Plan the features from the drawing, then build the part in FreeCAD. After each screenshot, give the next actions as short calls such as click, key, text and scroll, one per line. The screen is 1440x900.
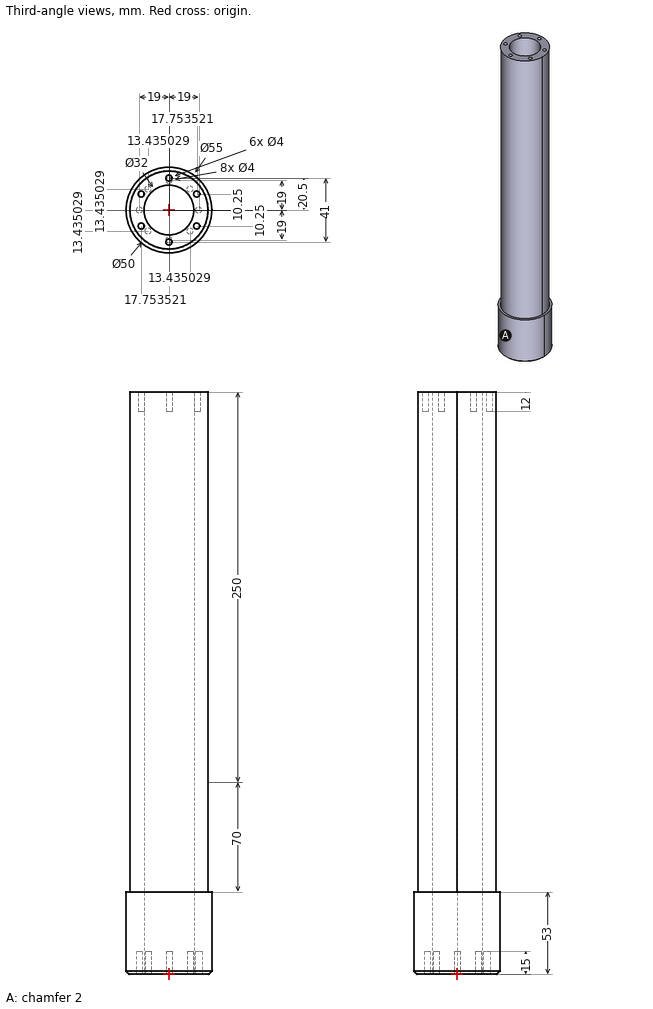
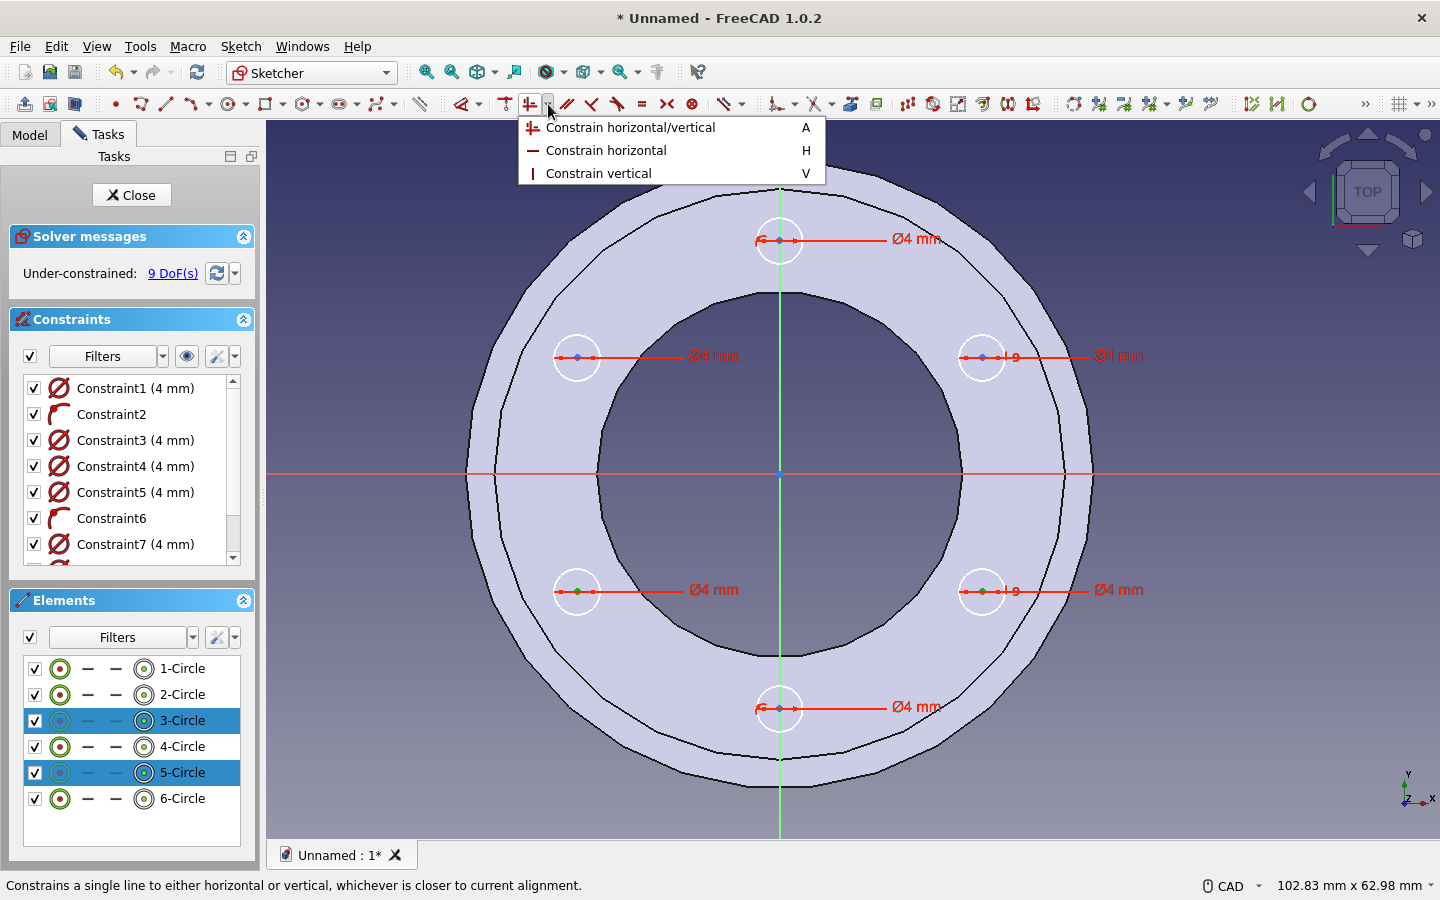
click(672, 150)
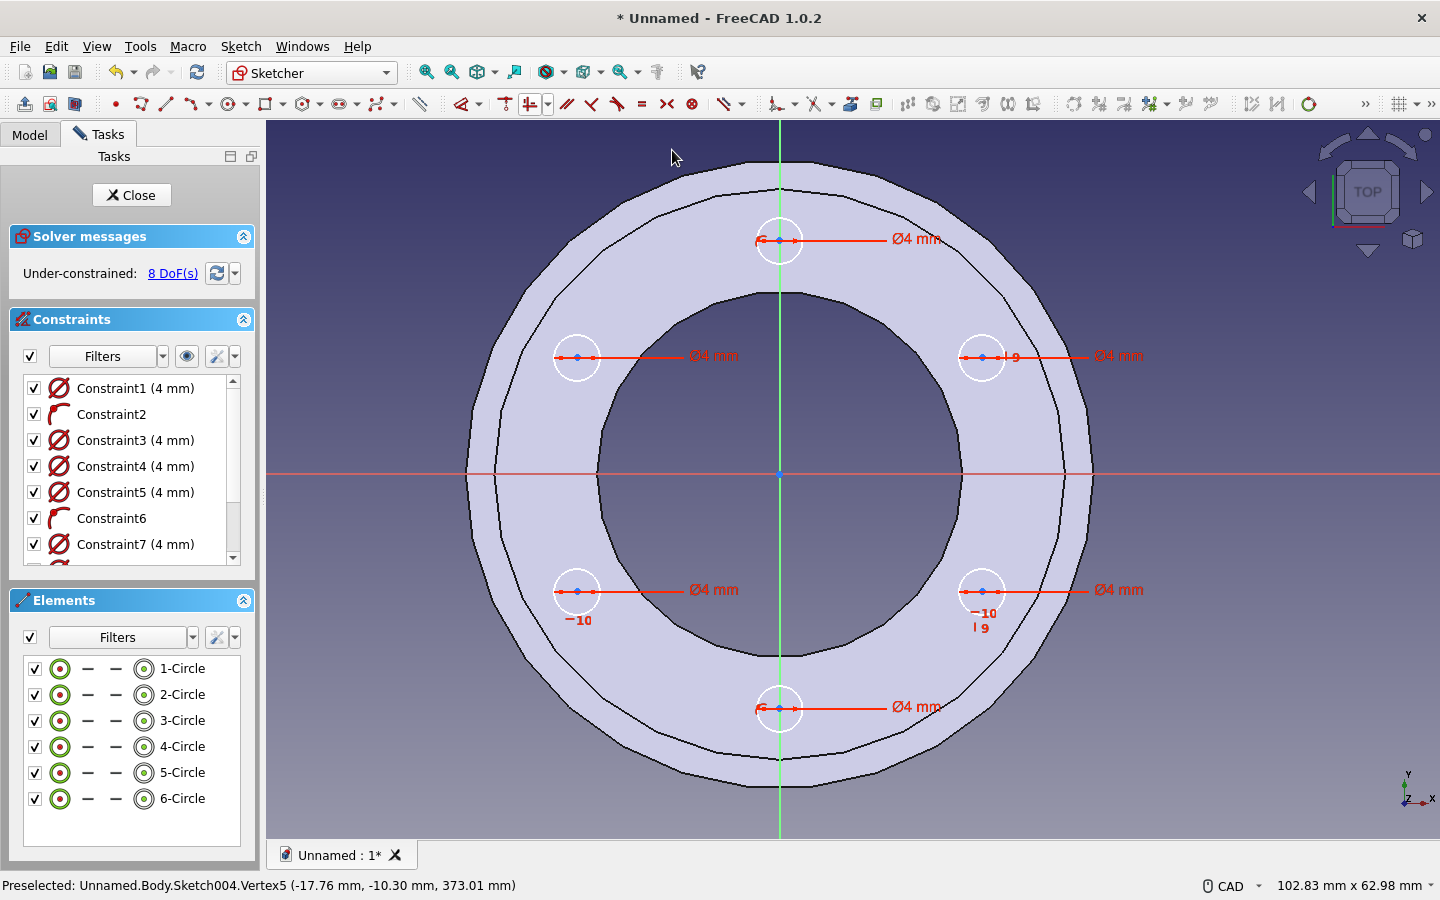
click(577, 592)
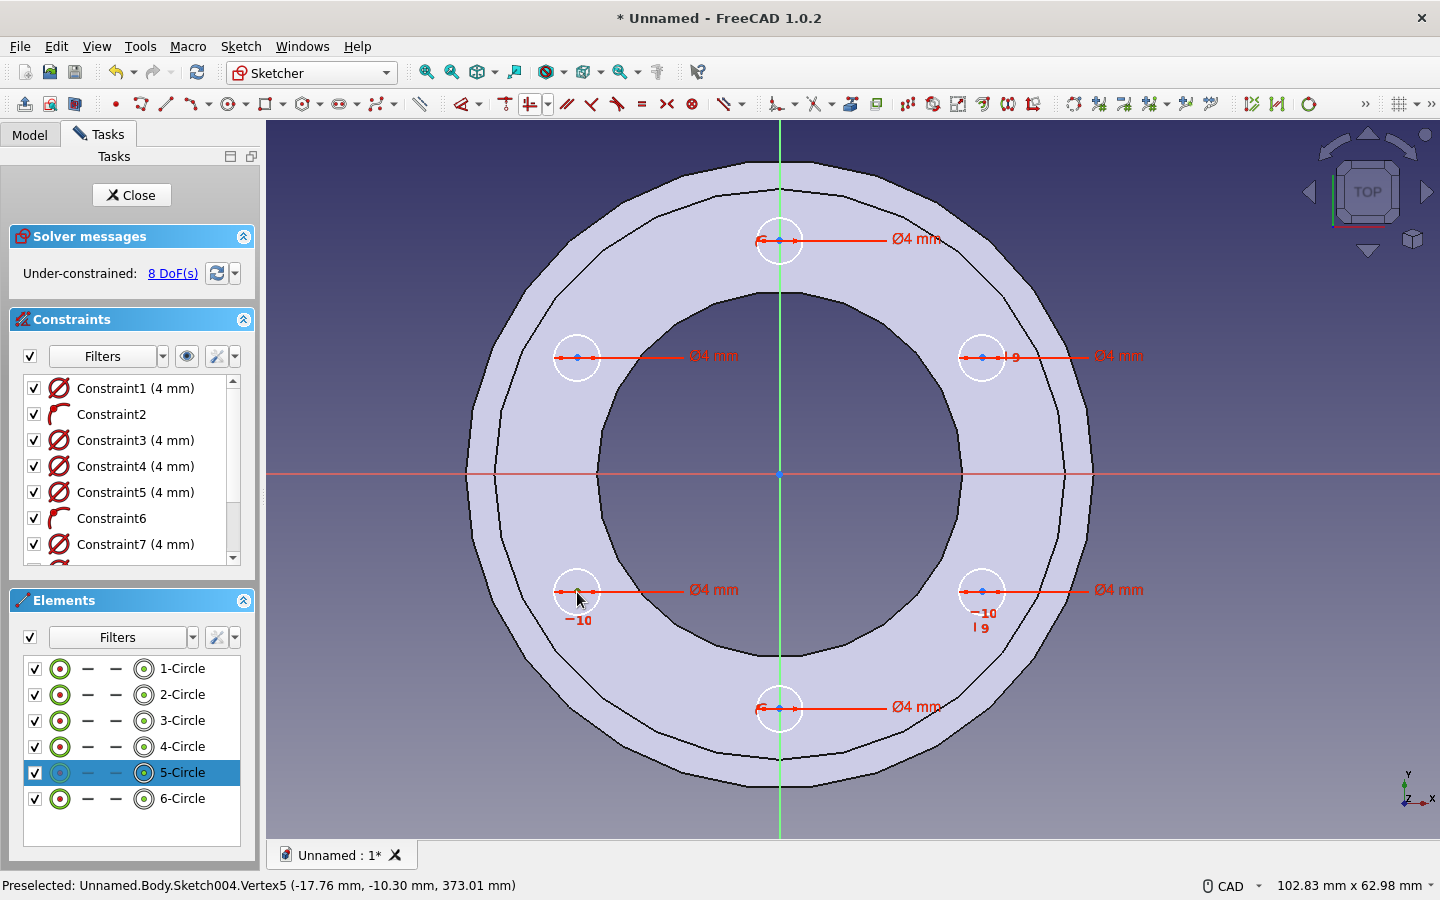
click(577, 358)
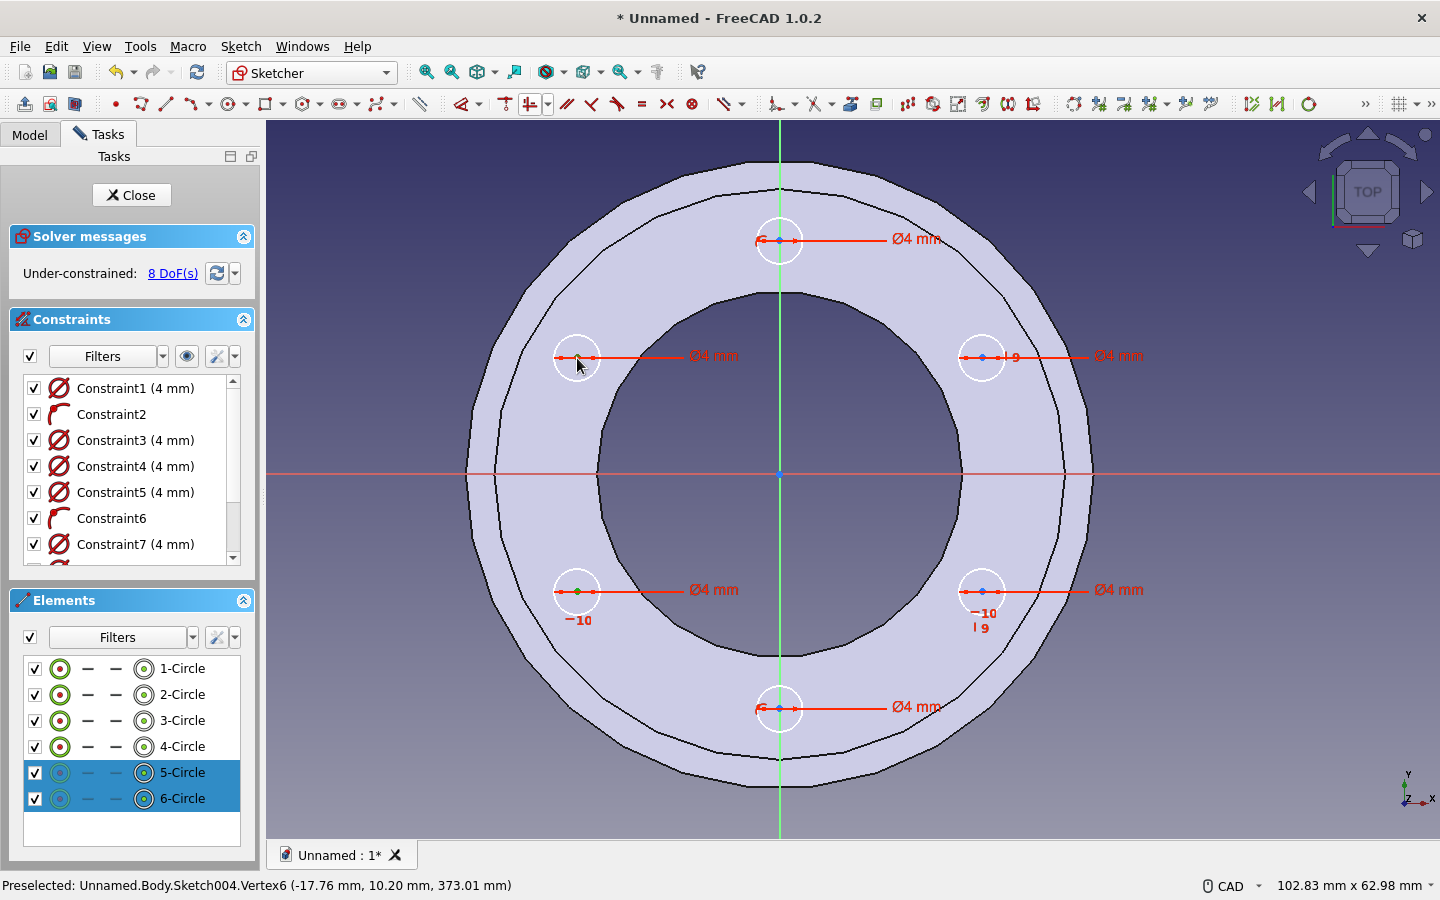
key(v)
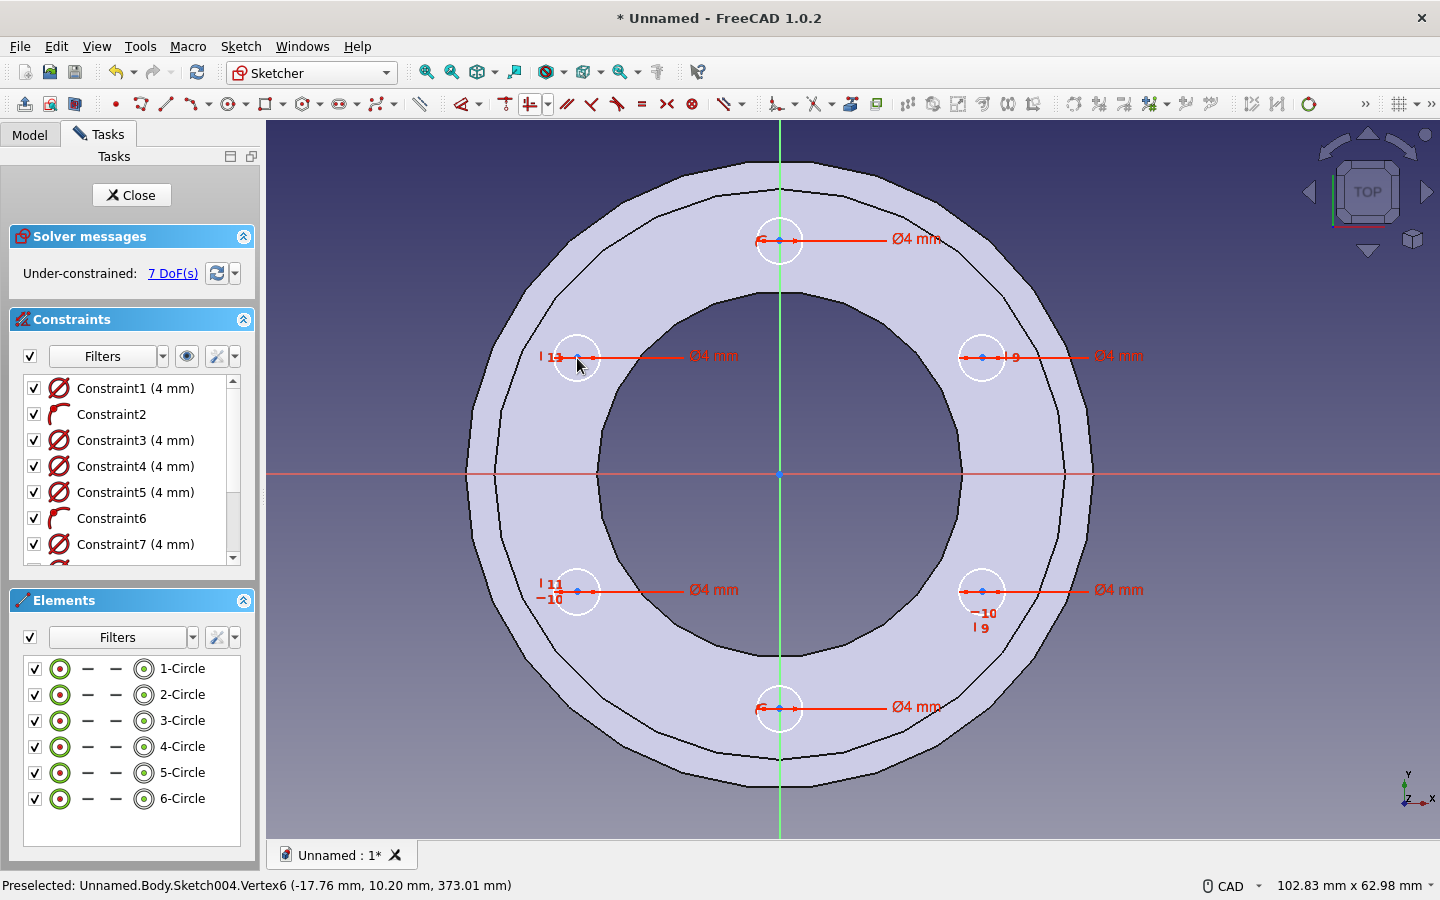
click(982, 358)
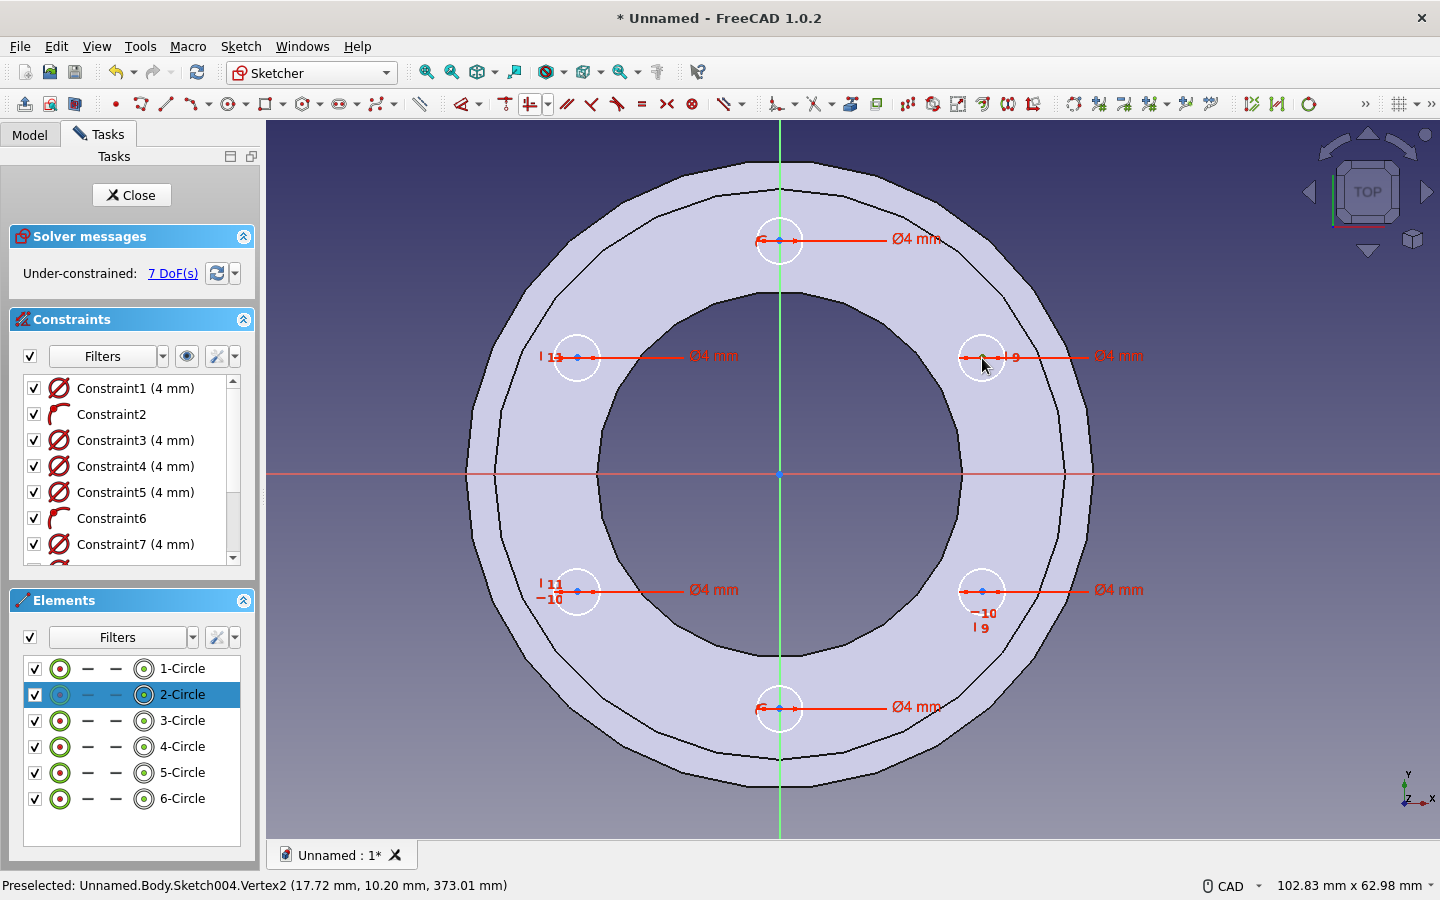
click(577, 358)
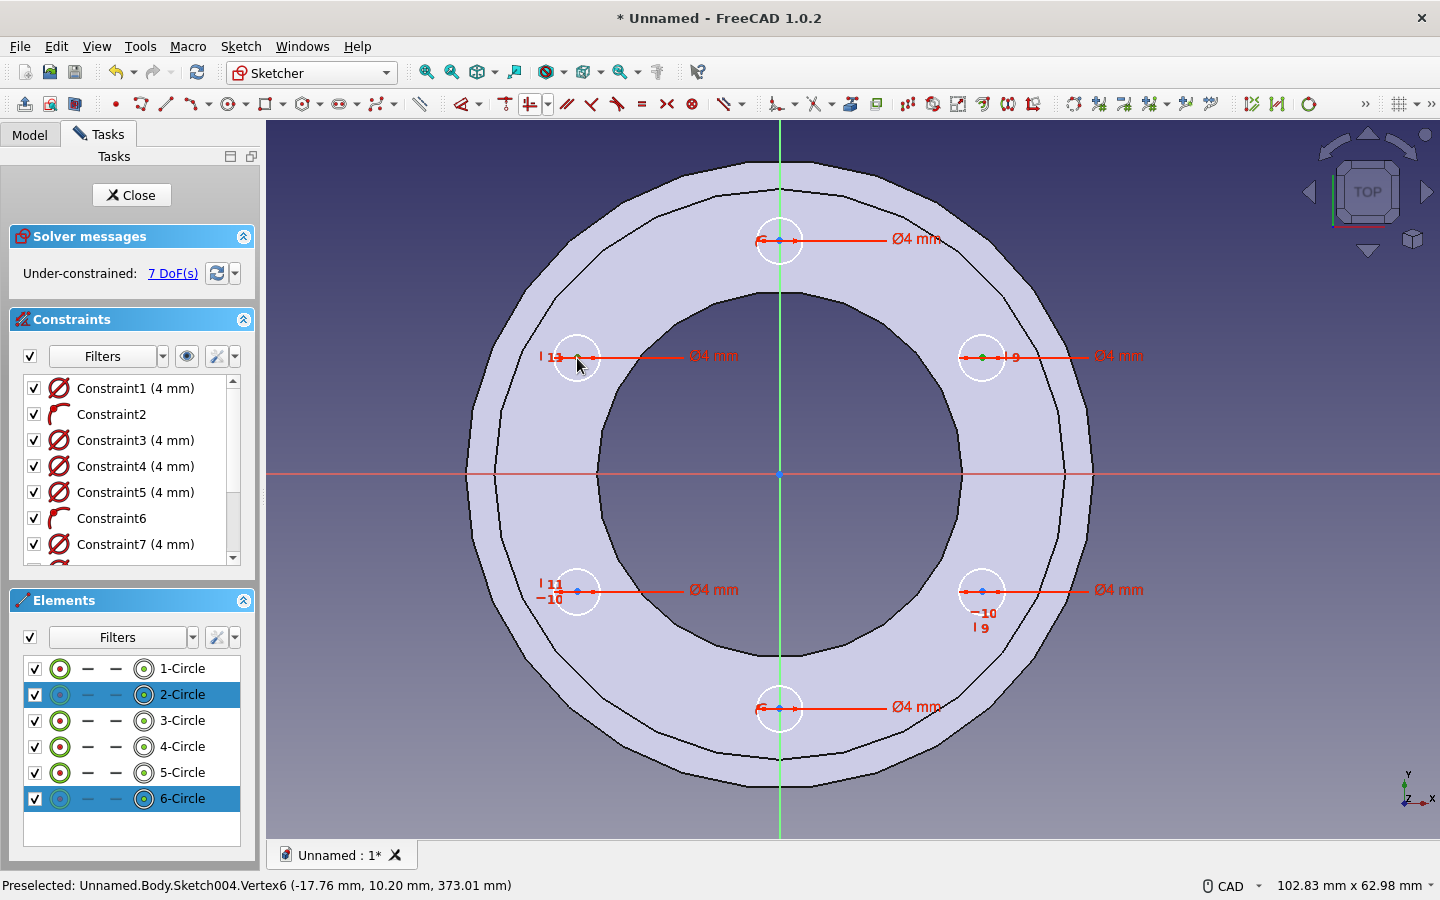
key(h)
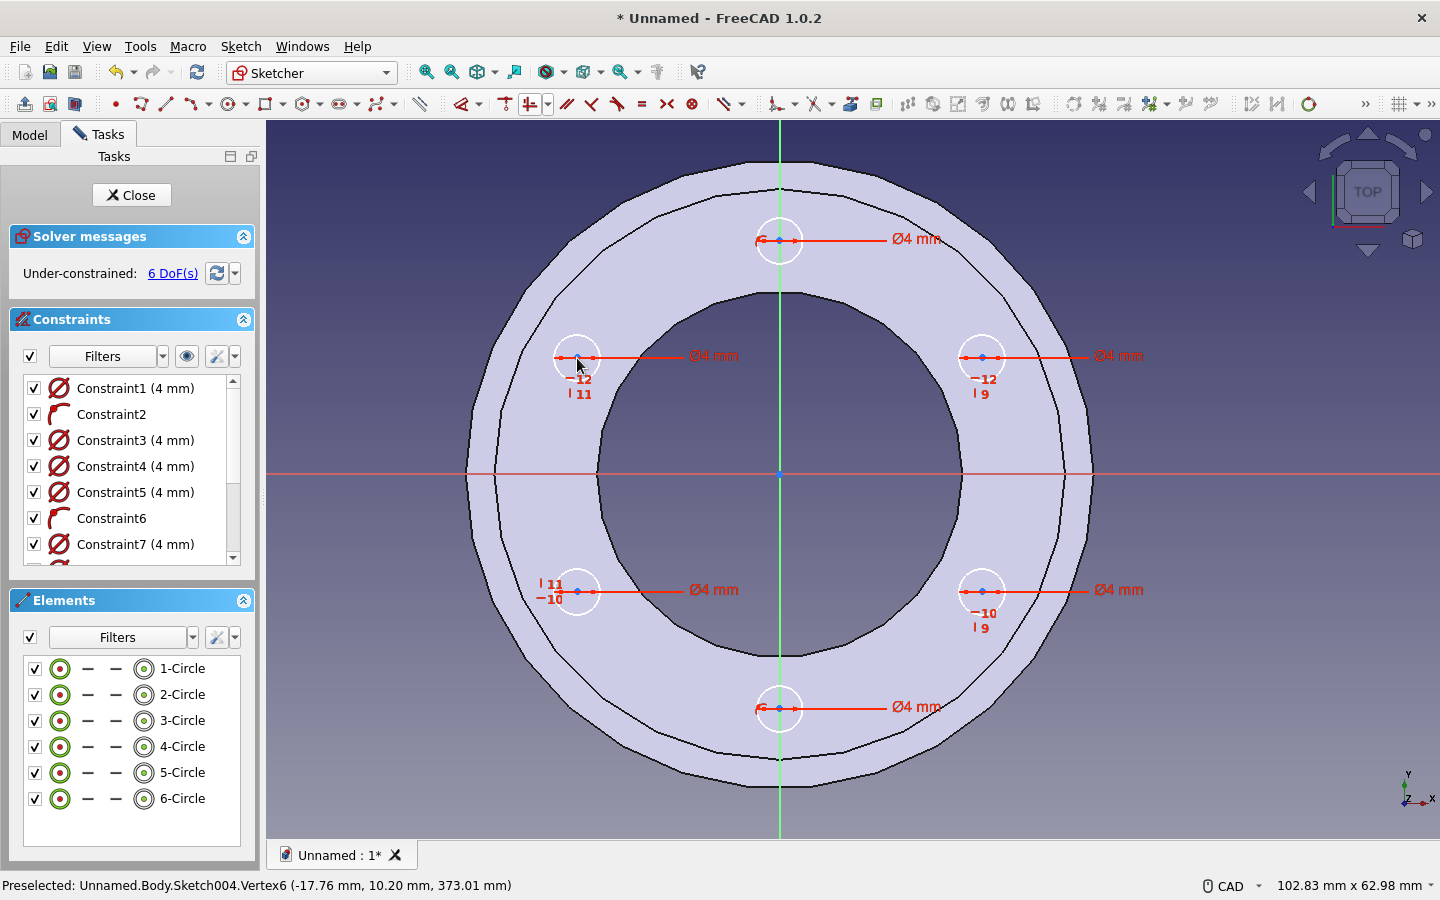
click(460, 104)